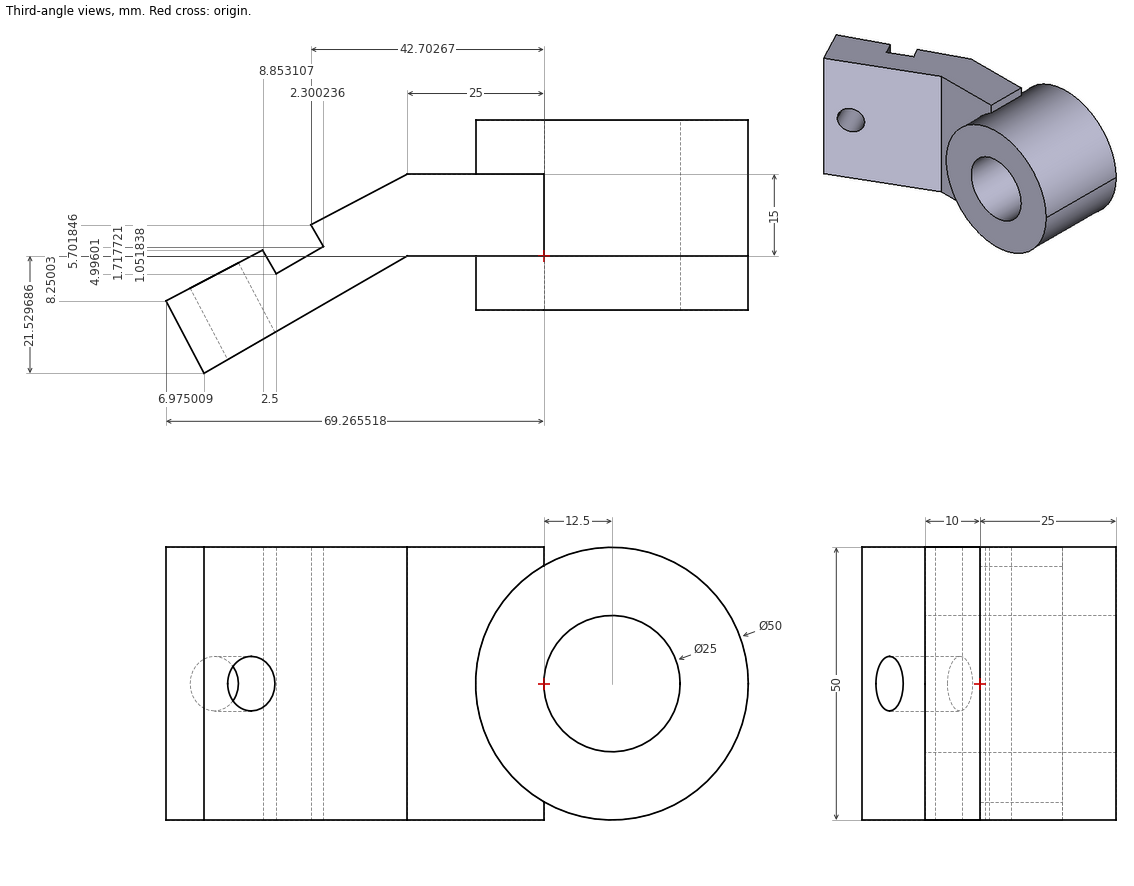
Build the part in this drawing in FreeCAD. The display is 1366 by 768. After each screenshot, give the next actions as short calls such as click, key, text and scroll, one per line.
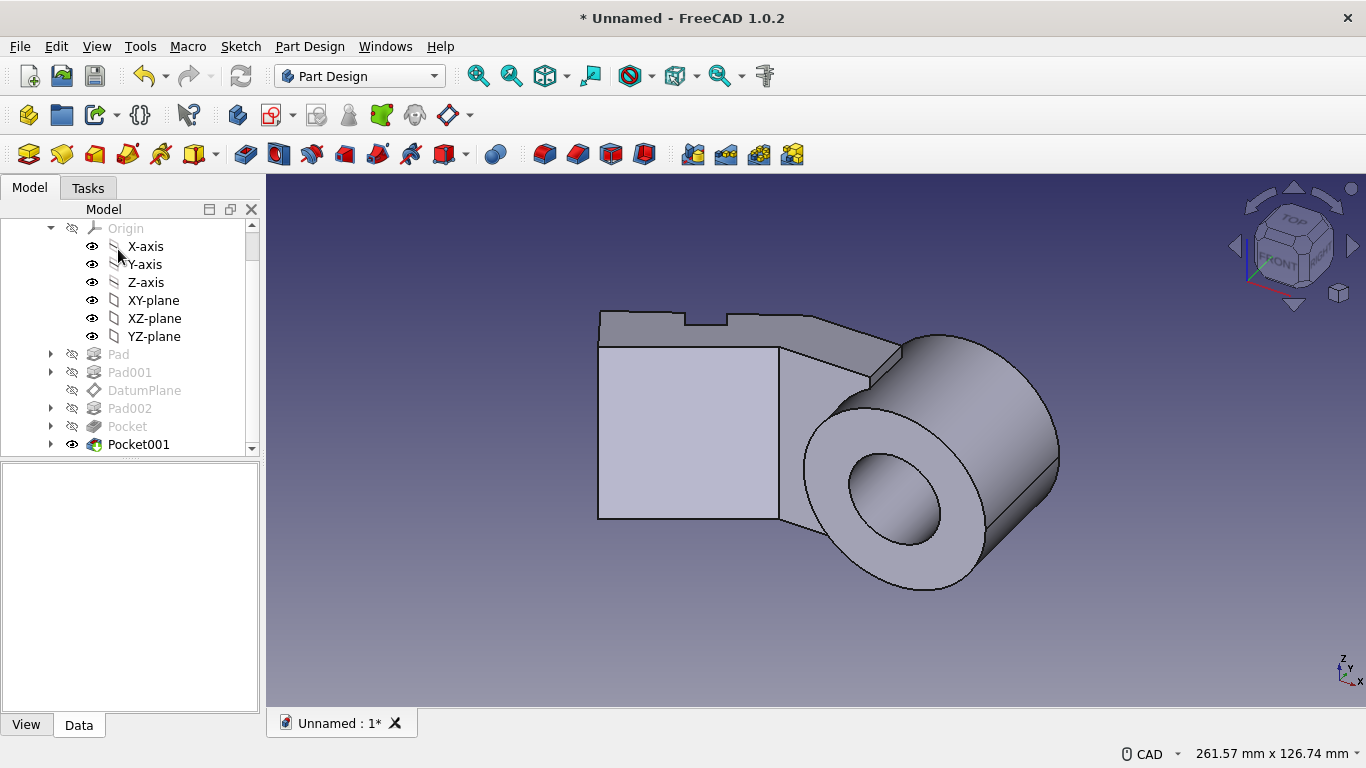
key(4)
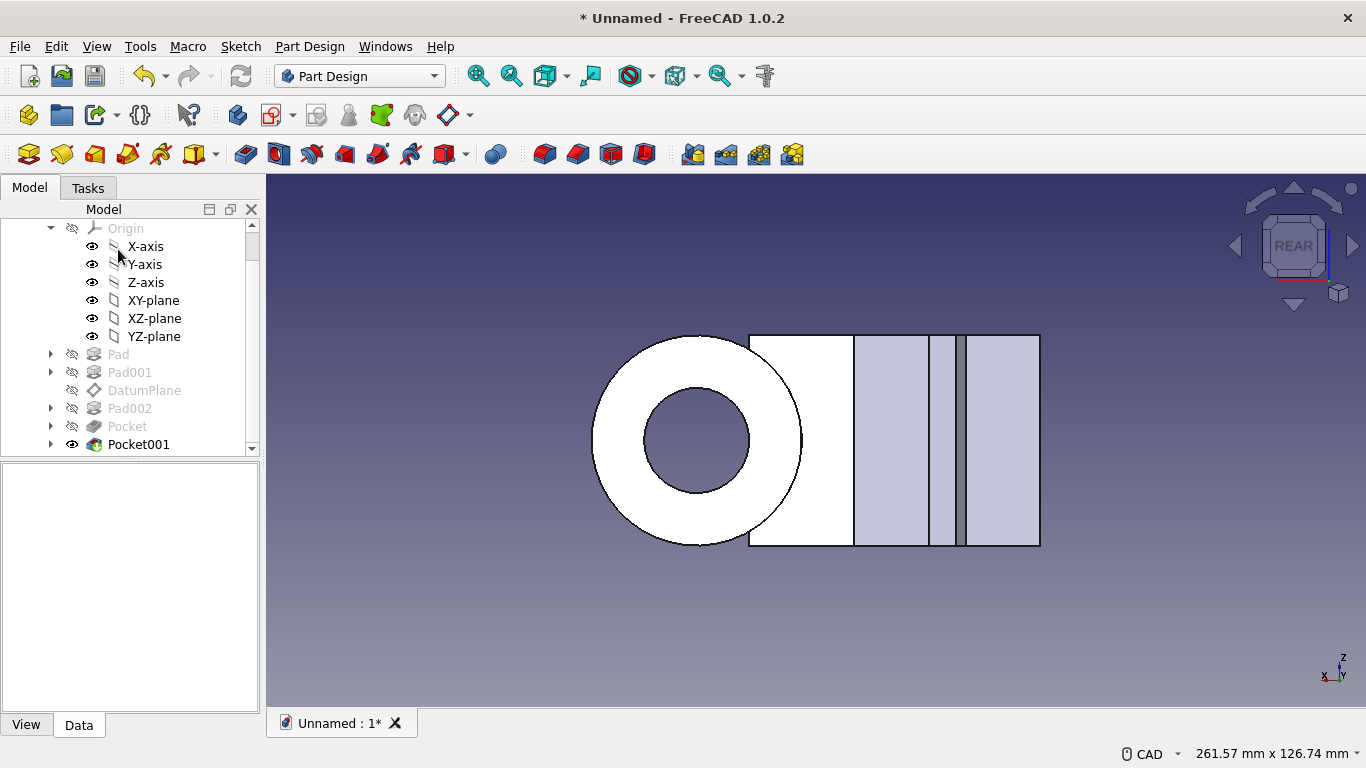
key(v)
key(f)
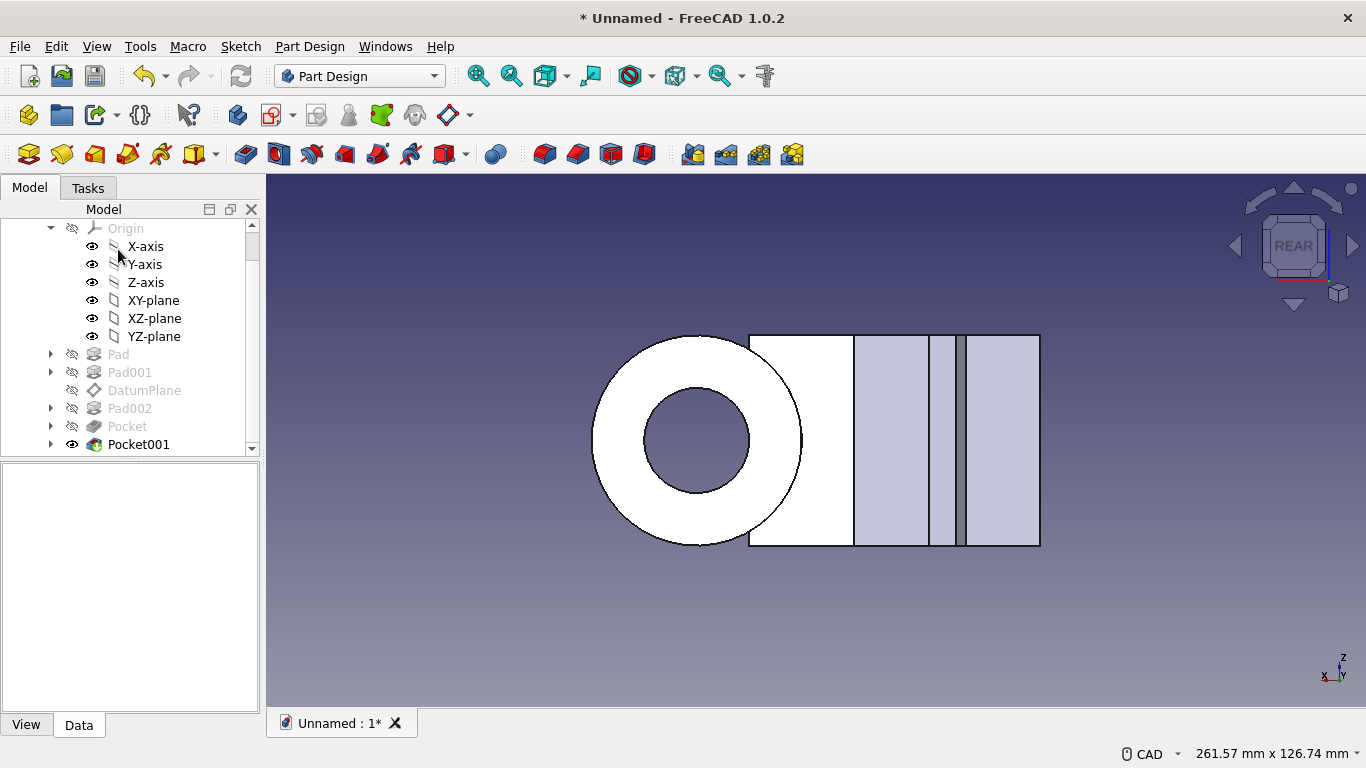
click(1003, 379)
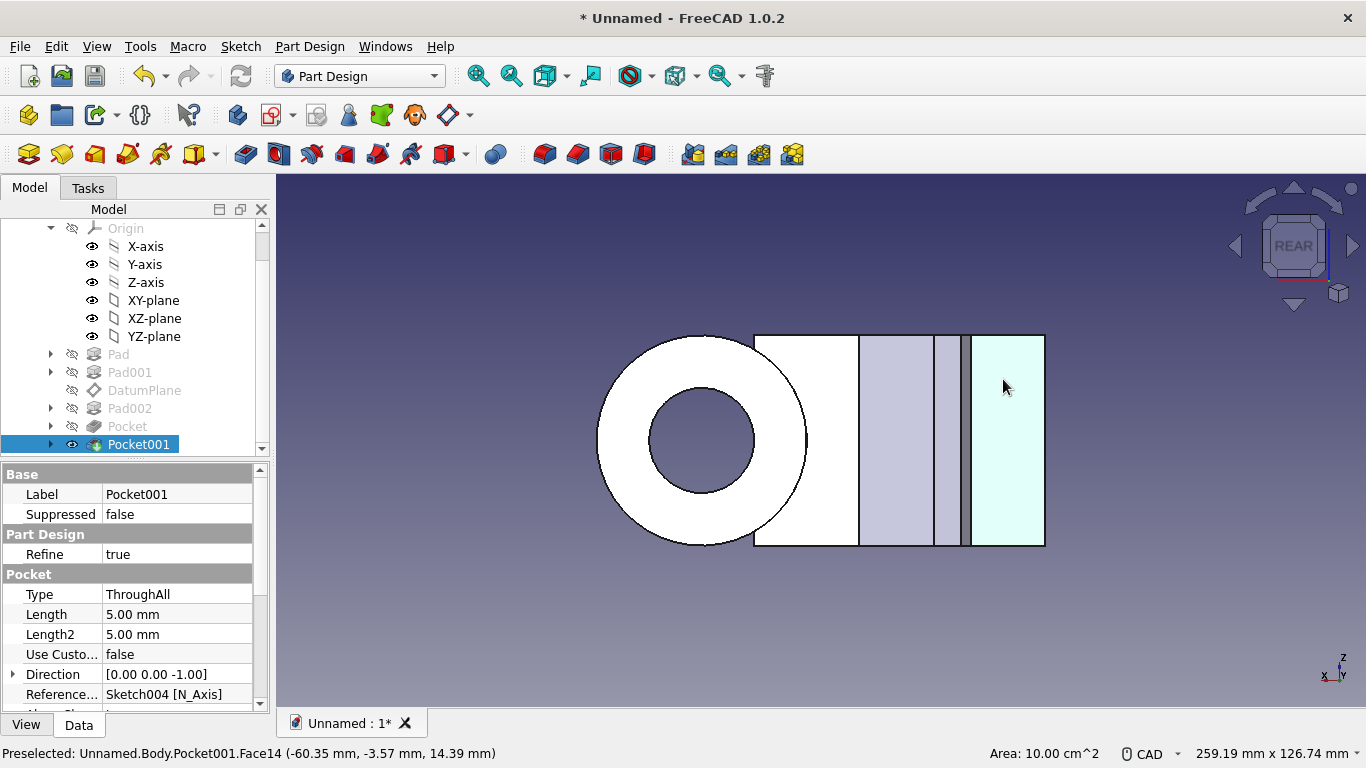
click(270, 116)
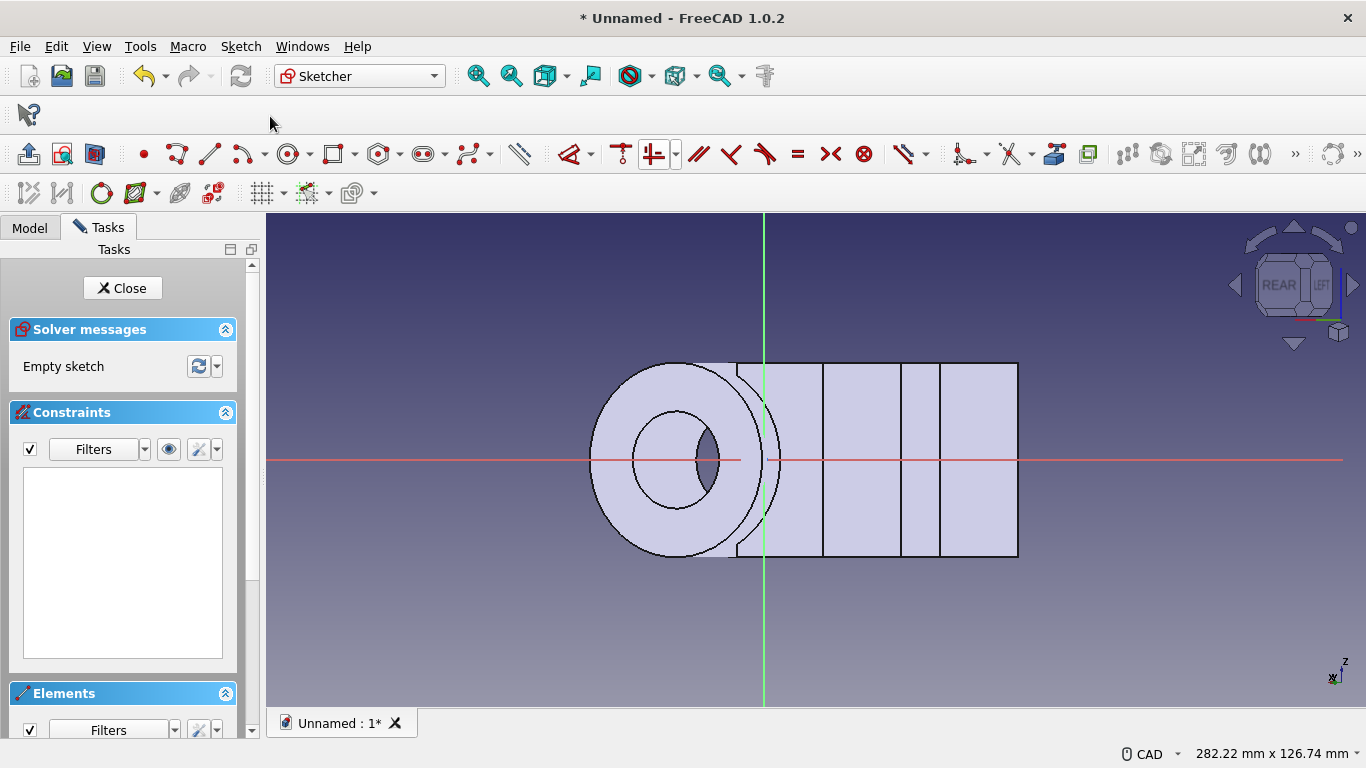
key(q)
key(s)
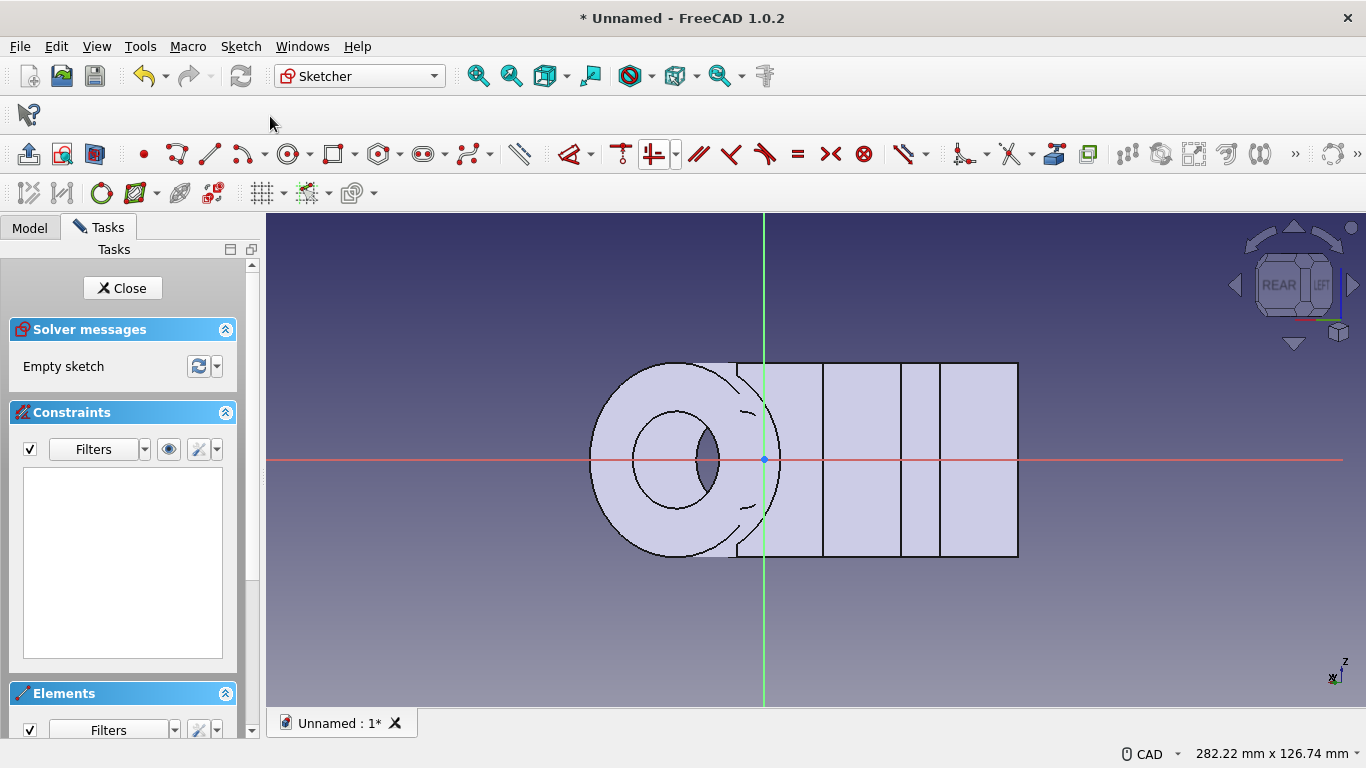
scroll(1016, 460, up, 10)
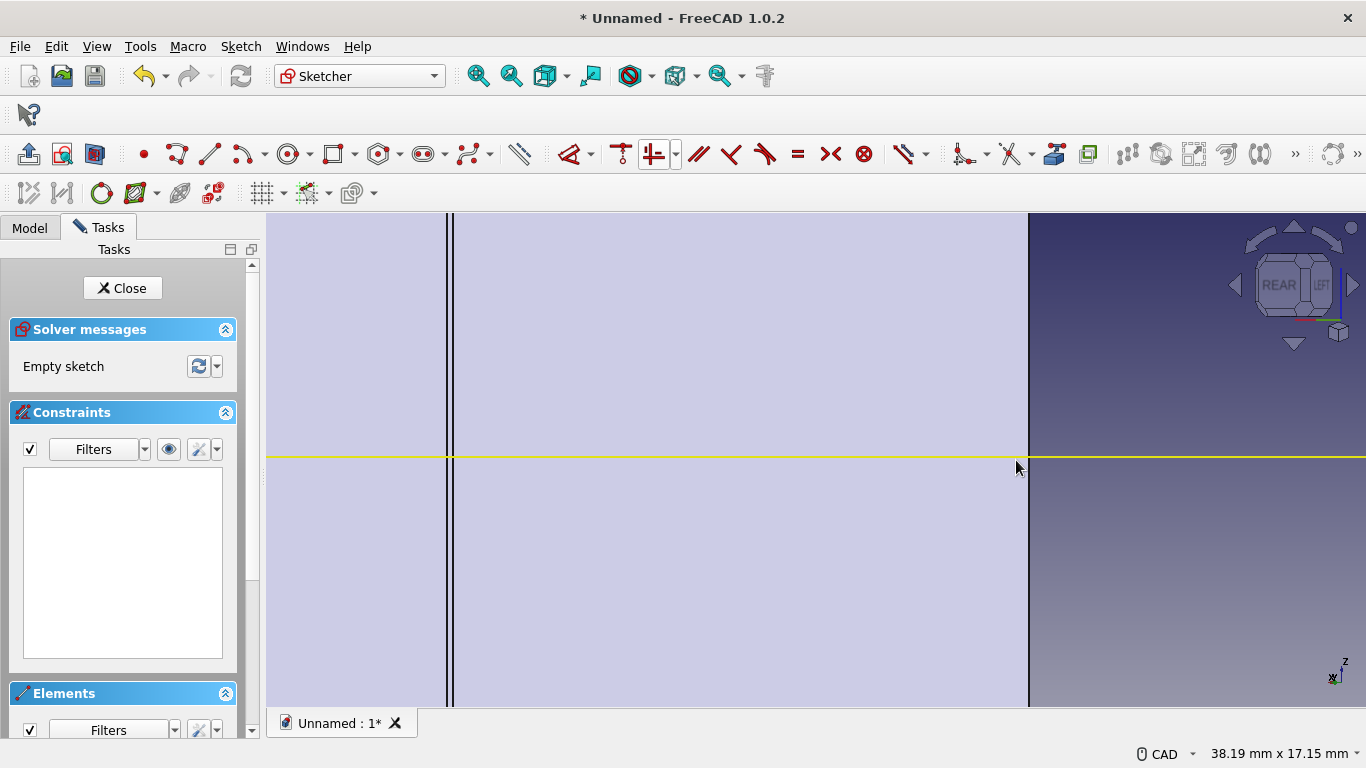
key(g)
key(c)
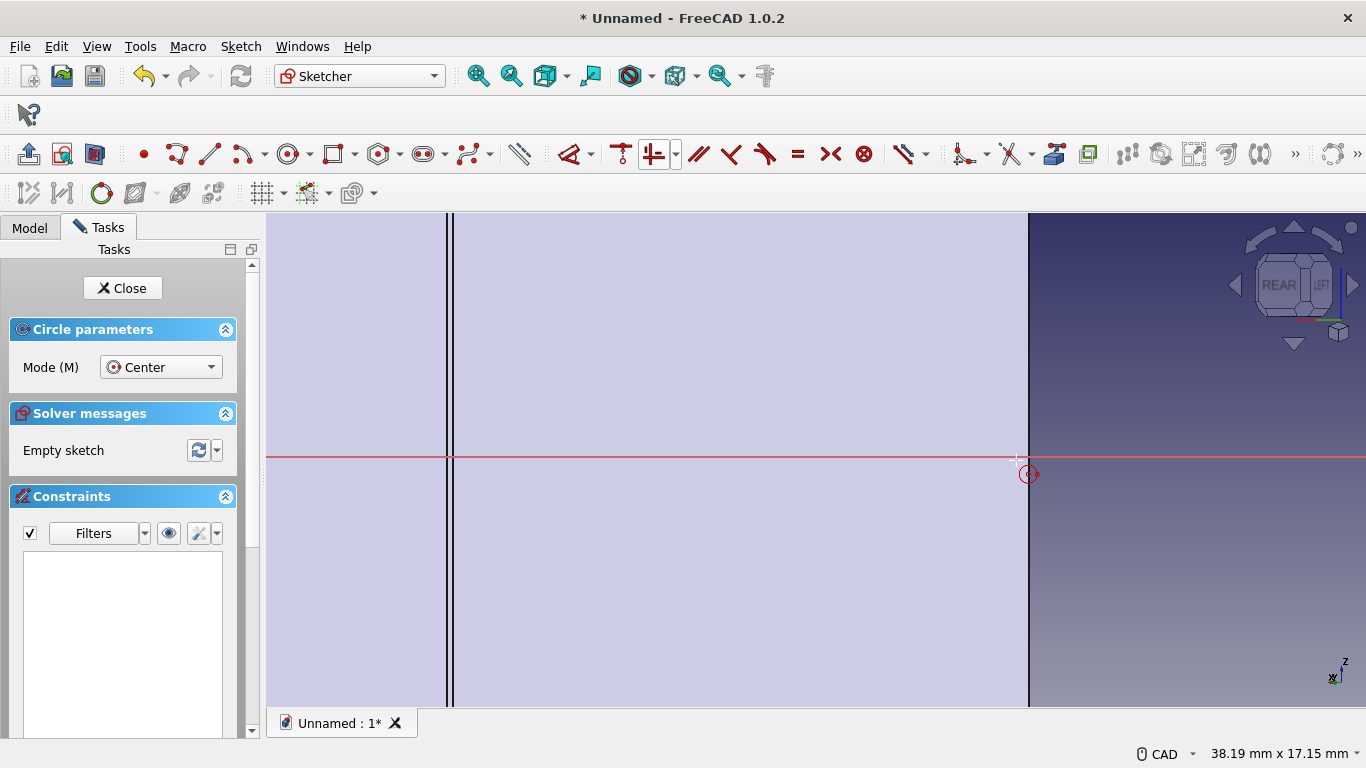
click(741, 457)
click(842, 355)
key(Escape)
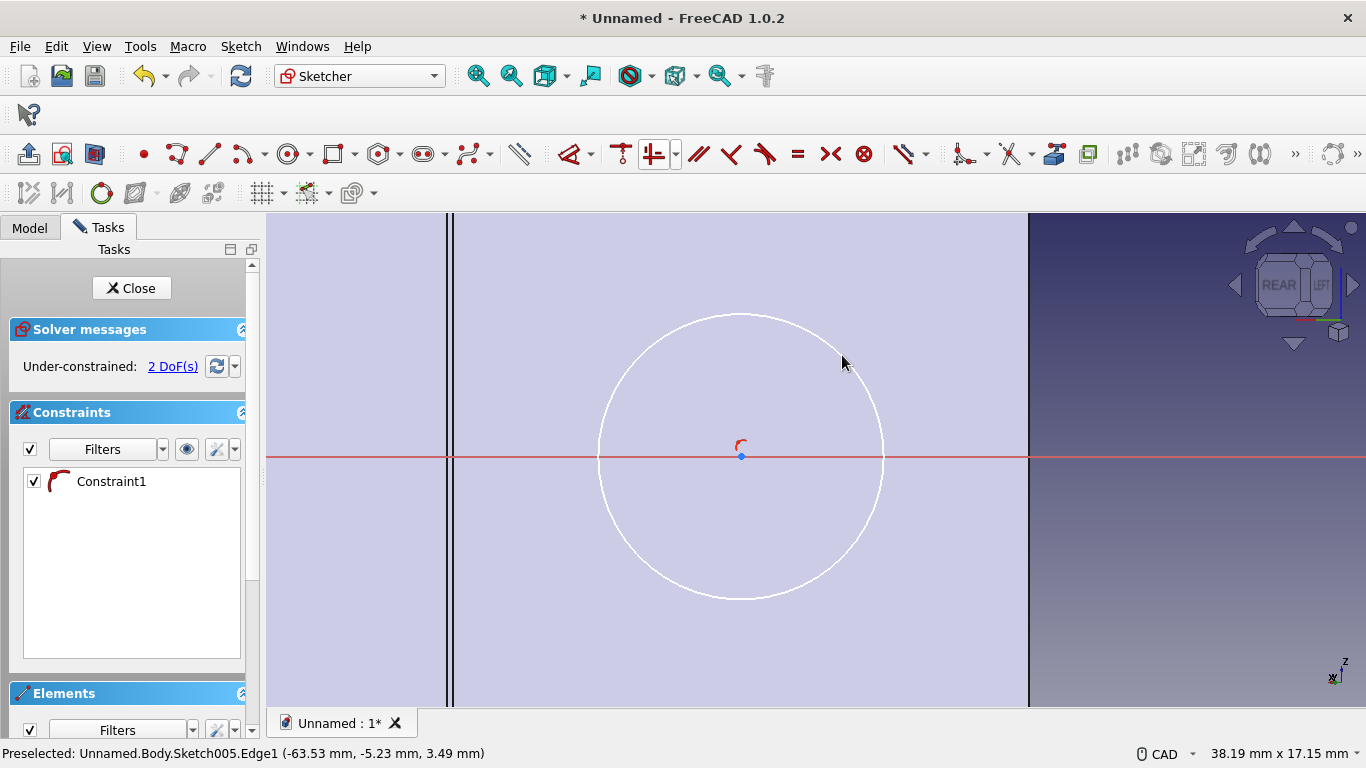
click(568, 154)